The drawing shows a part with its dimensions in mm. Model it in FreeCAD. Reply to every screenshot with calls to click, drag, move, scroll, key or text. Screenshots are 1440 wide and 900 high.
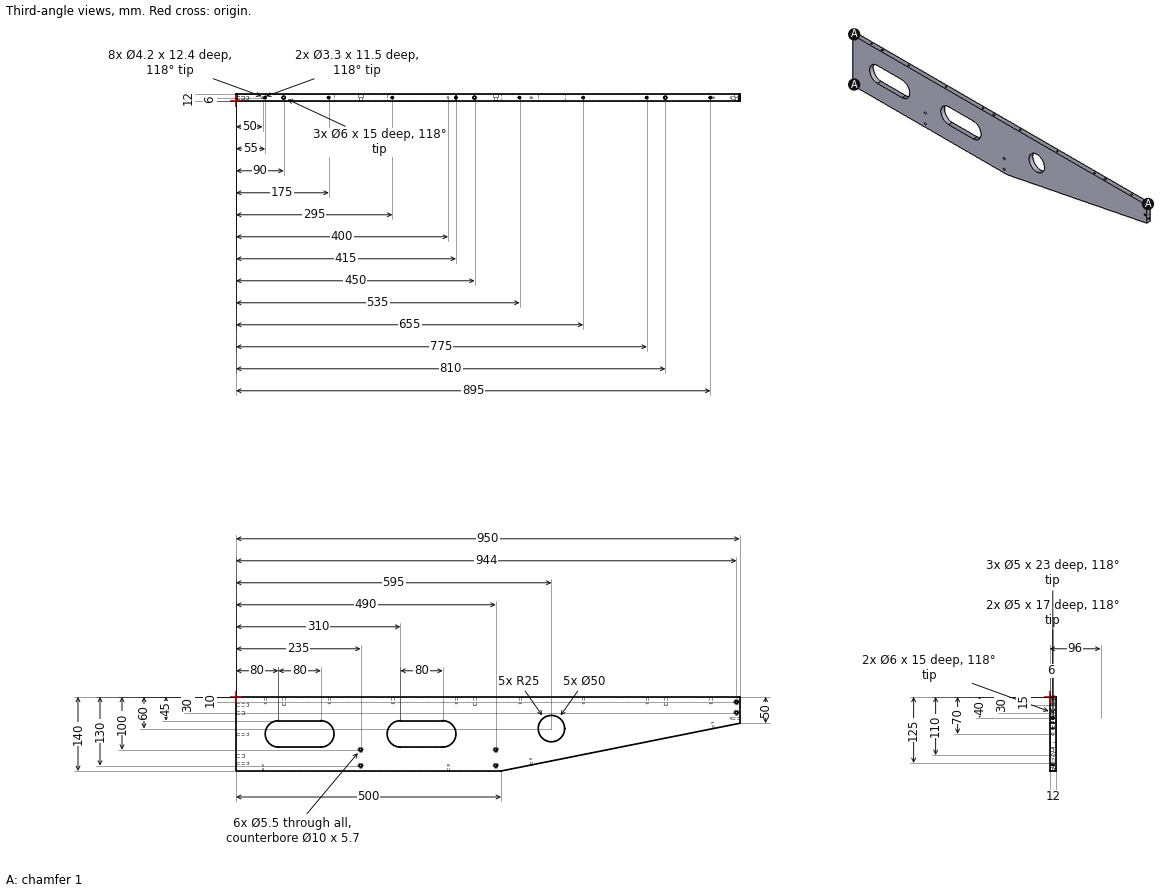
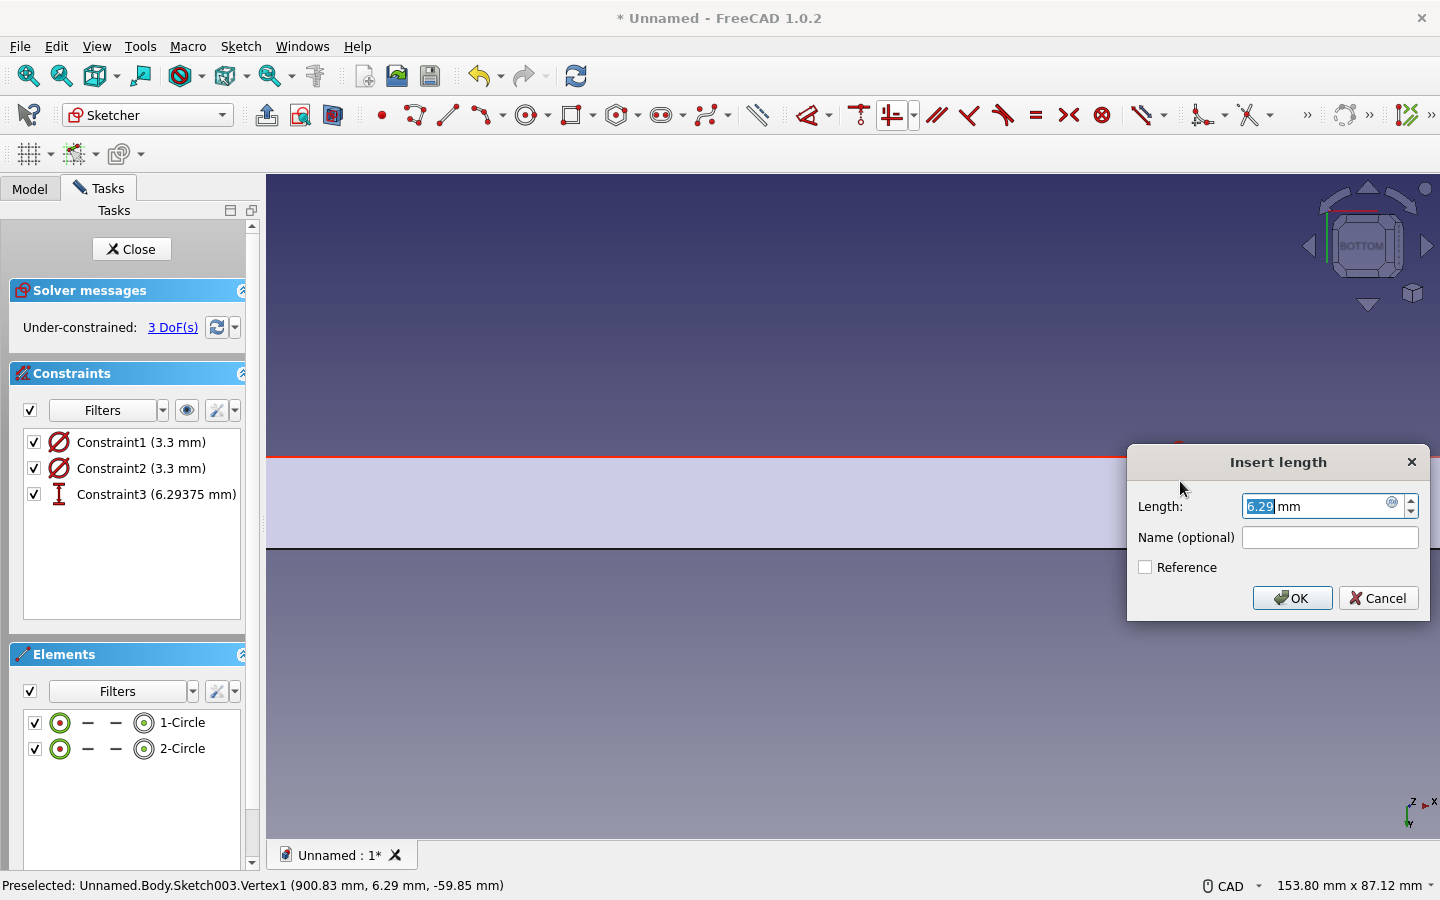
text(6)
key(Return)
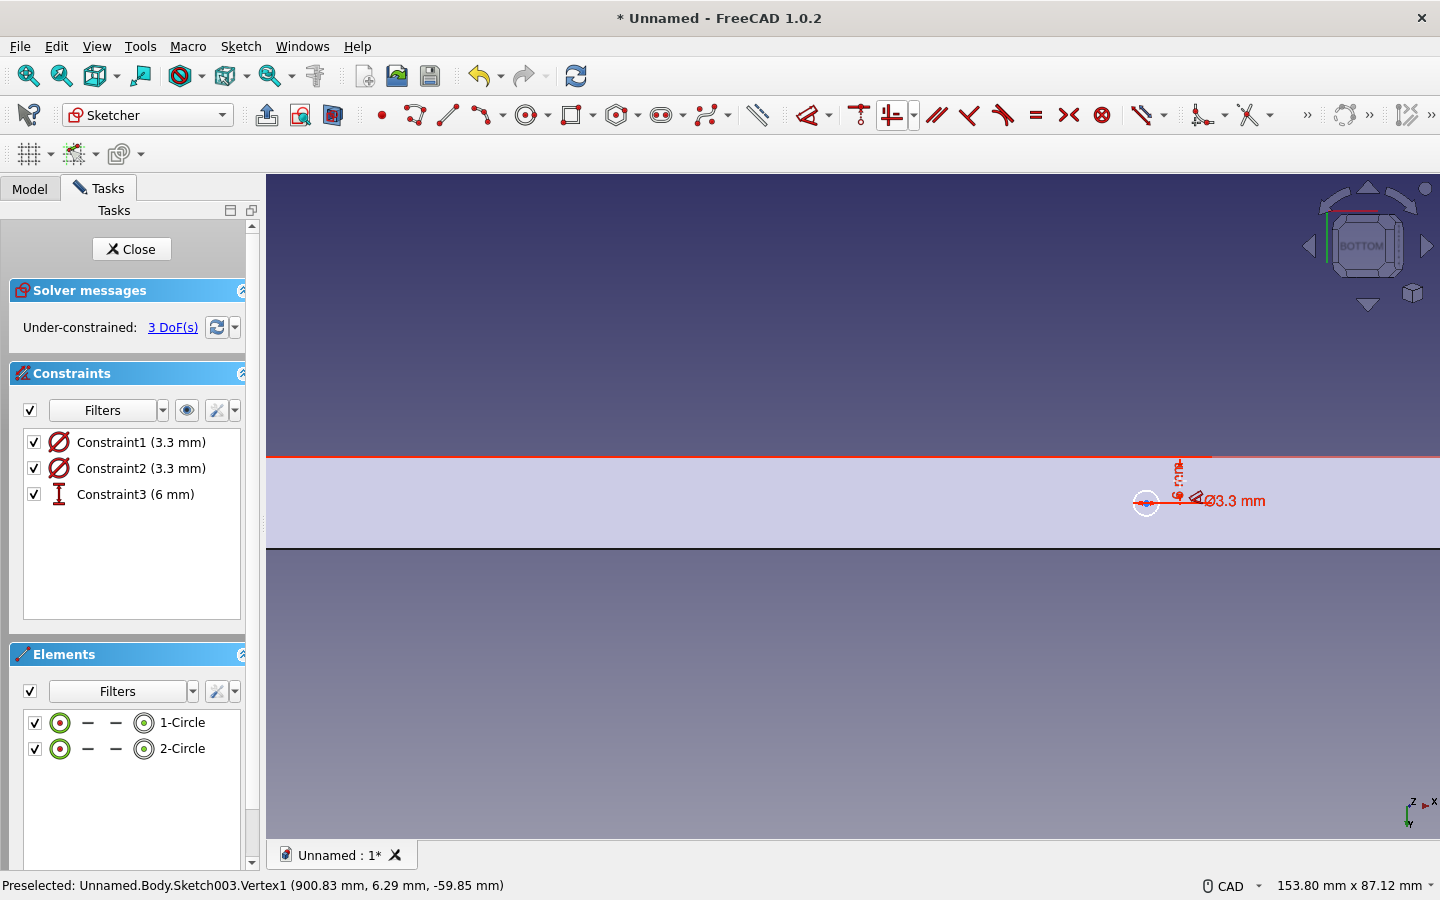
scroll(1153, 509, down, 11)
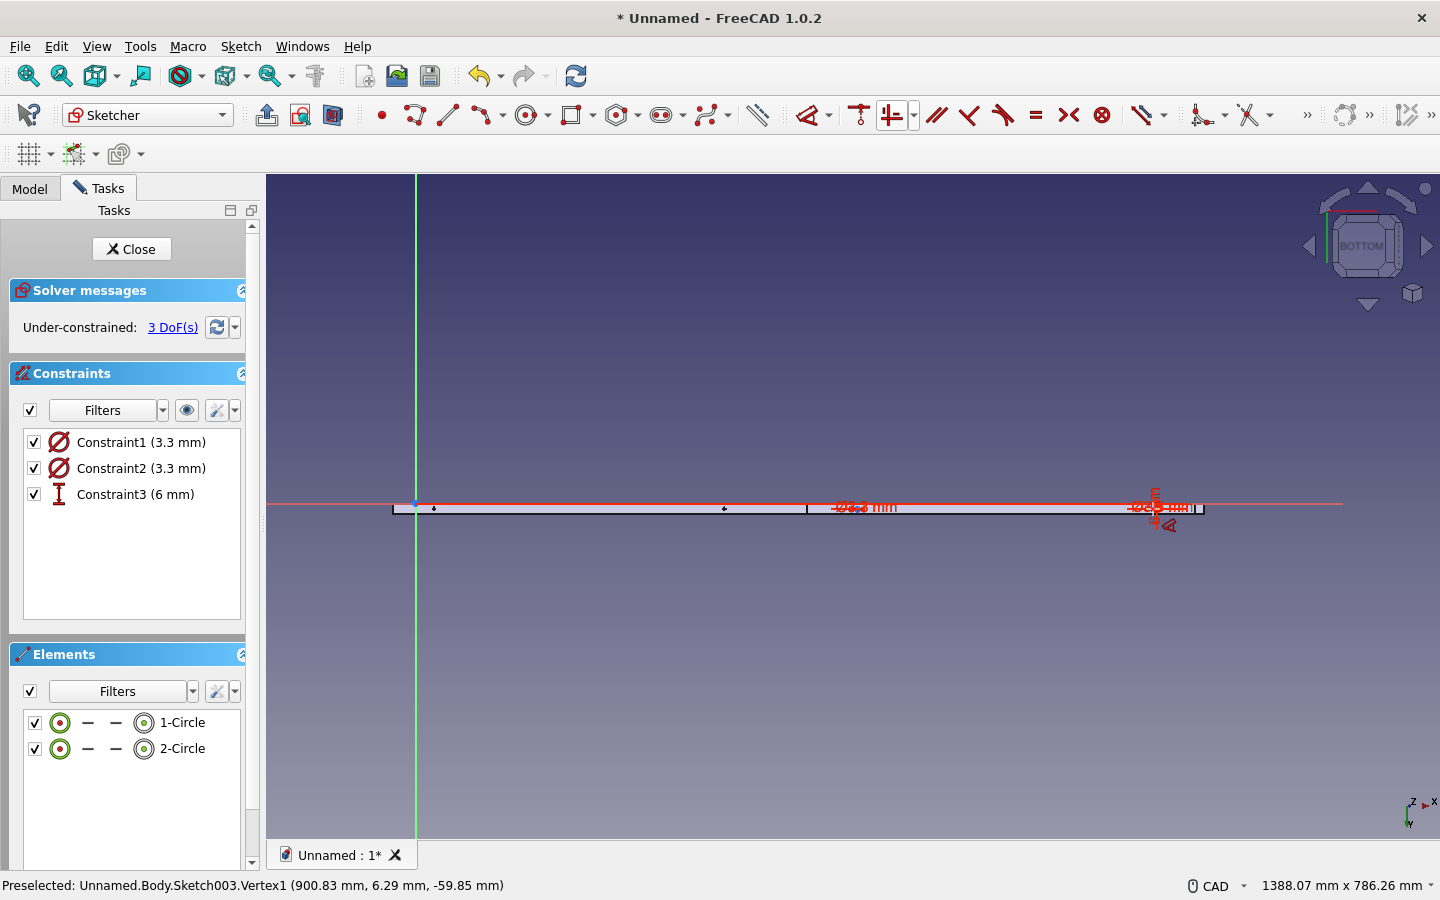
scroll(857, 509, up, 11)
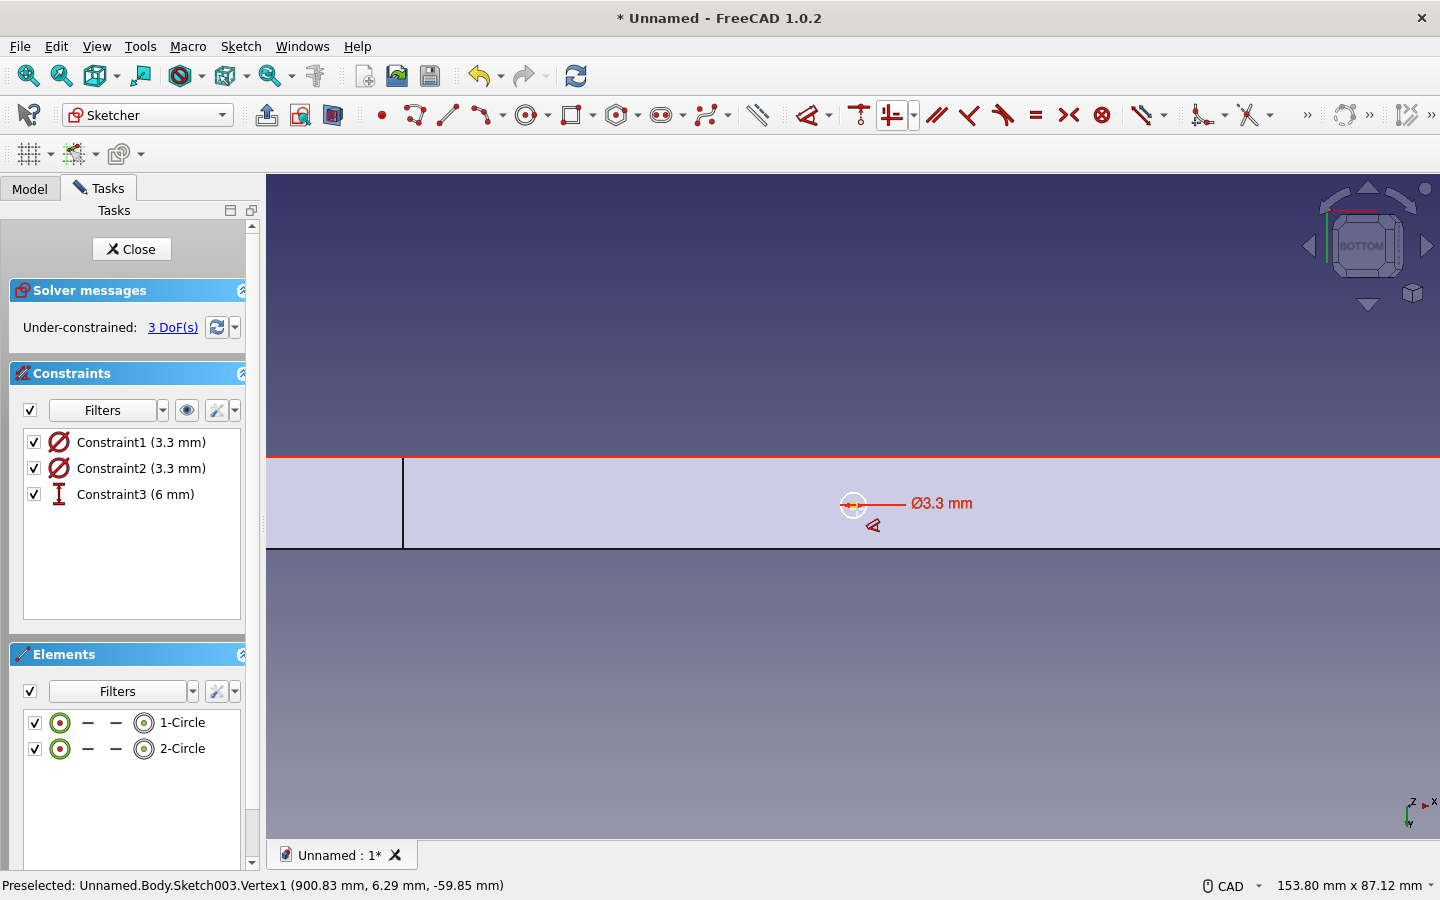
click(853, 505)
click(887, 481)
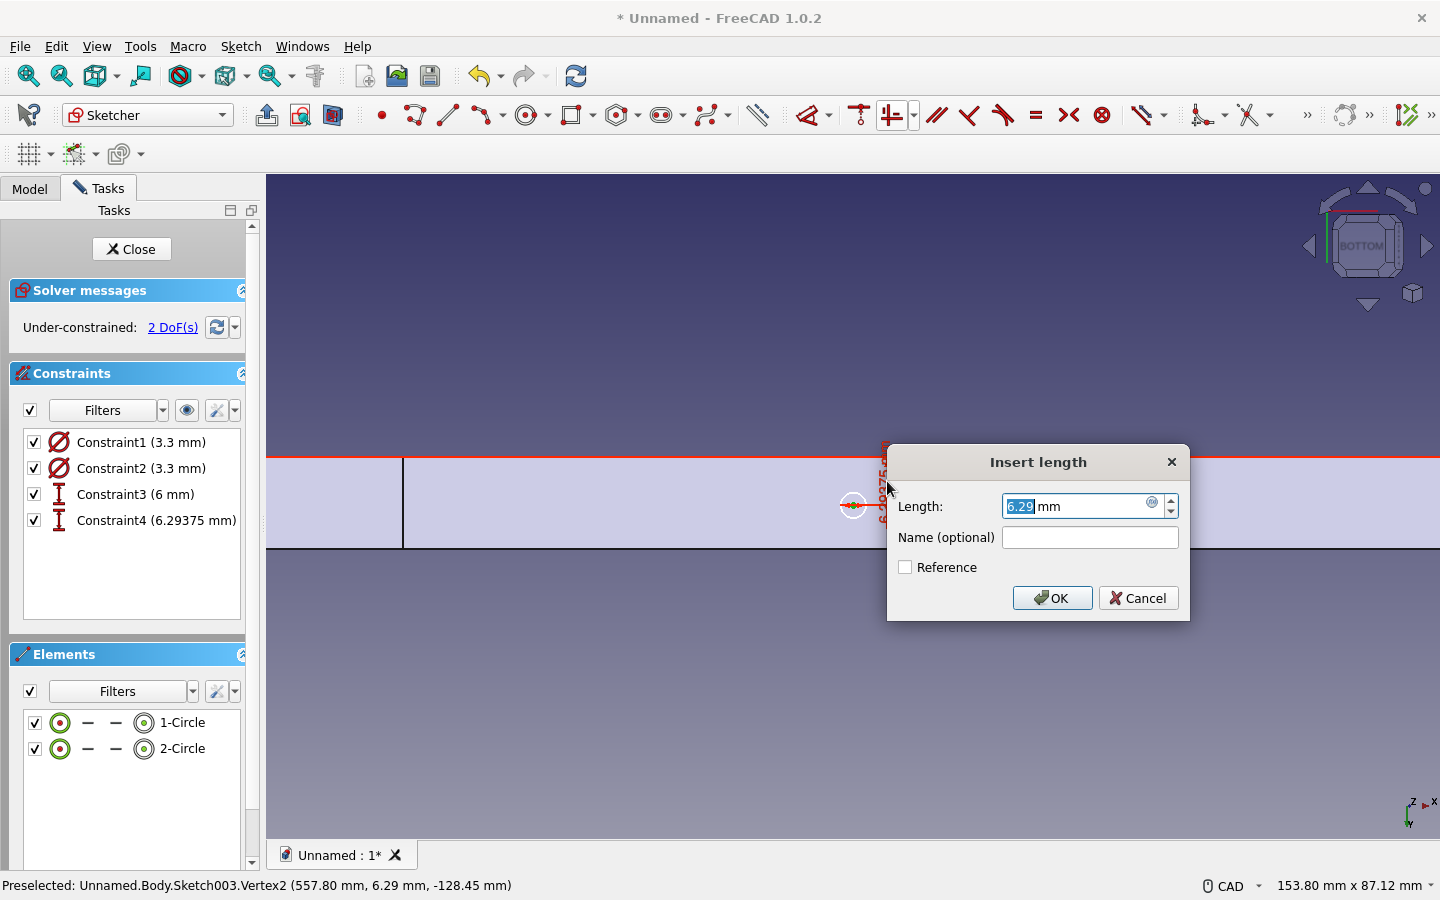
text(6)
key(Return)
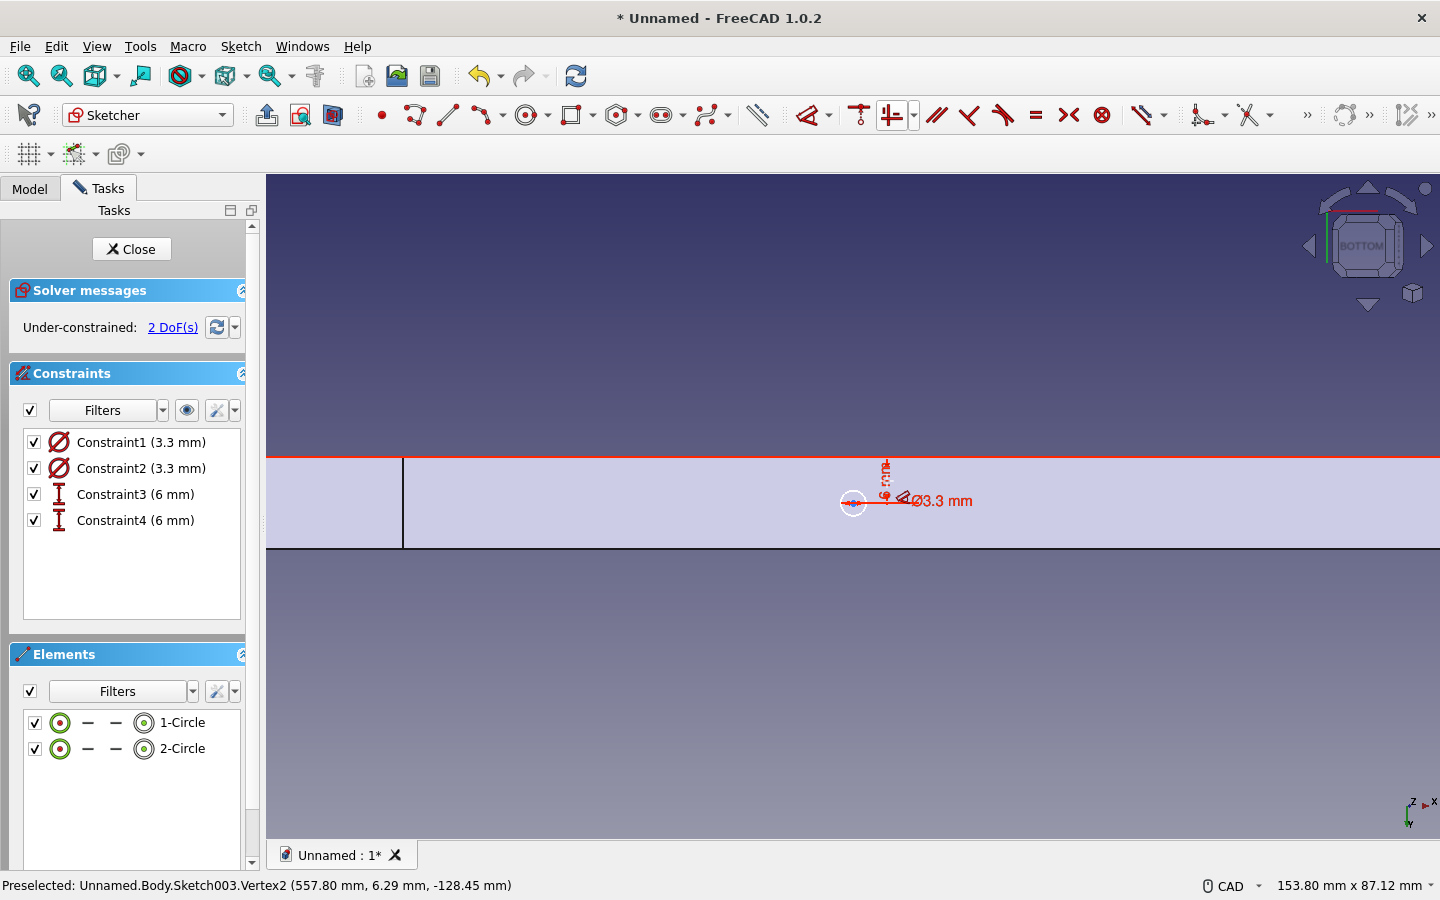
scroll(857, 509, down, 11)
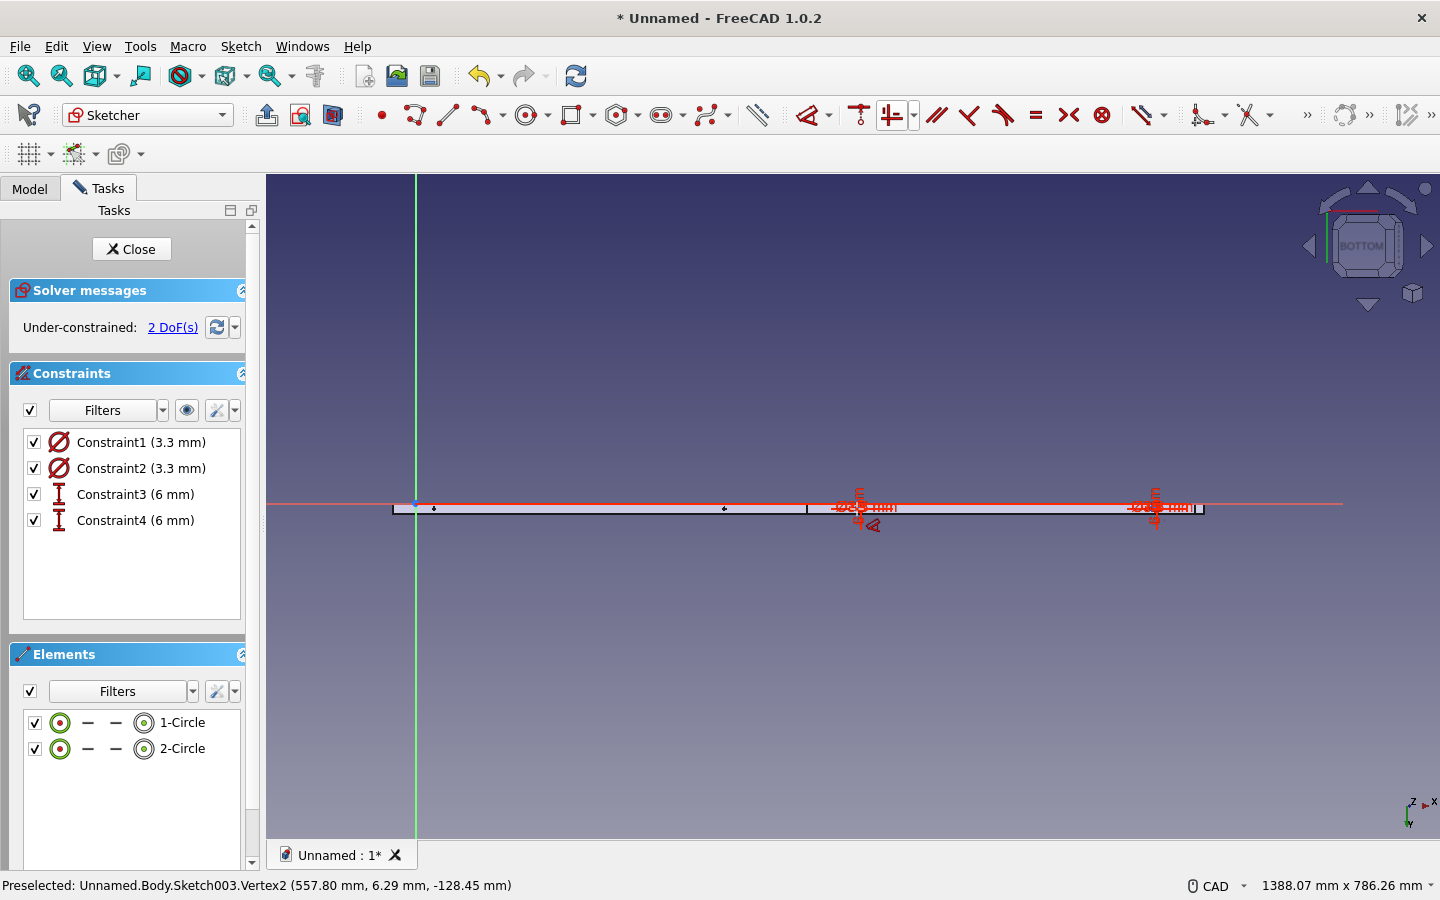
click(1153, 509)